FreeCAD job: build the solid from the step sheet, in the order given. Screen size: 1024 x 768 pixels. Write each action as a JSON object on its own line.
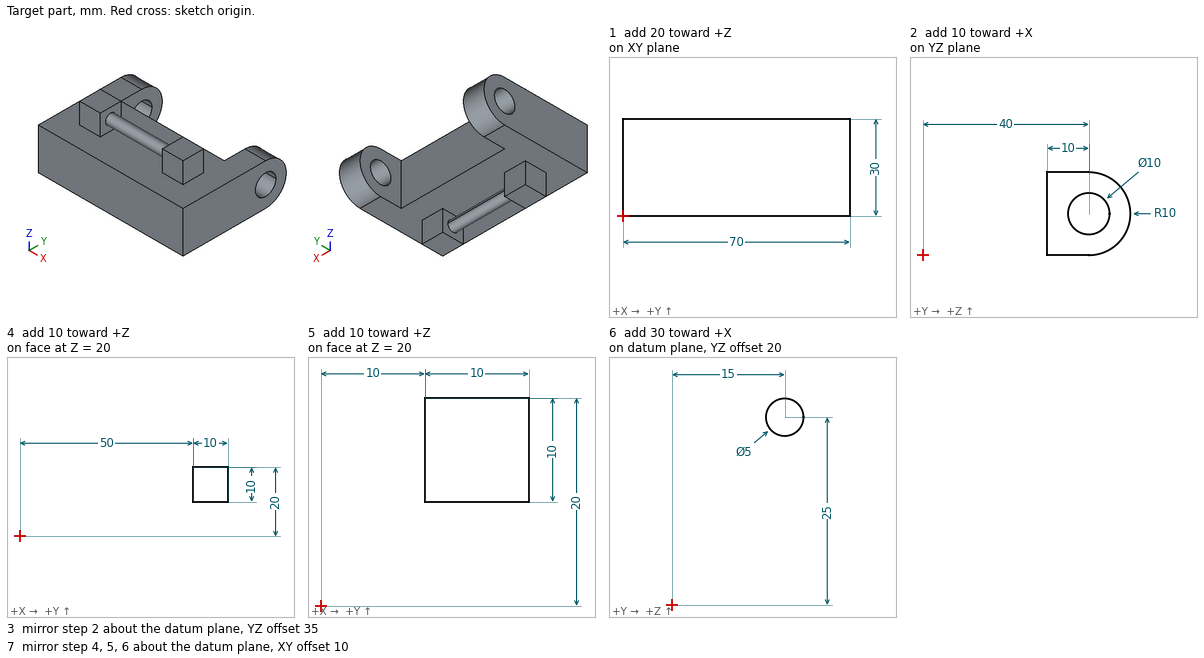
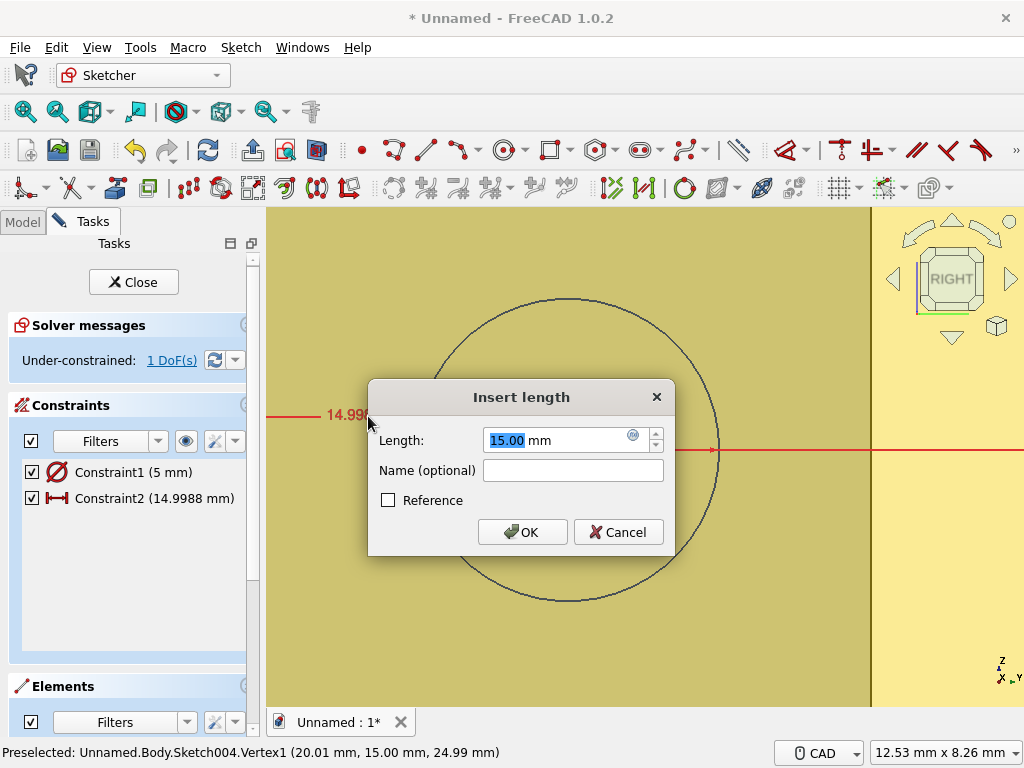
{"action": "type", "text": "15"}
{"action": "key", "text": "Return"}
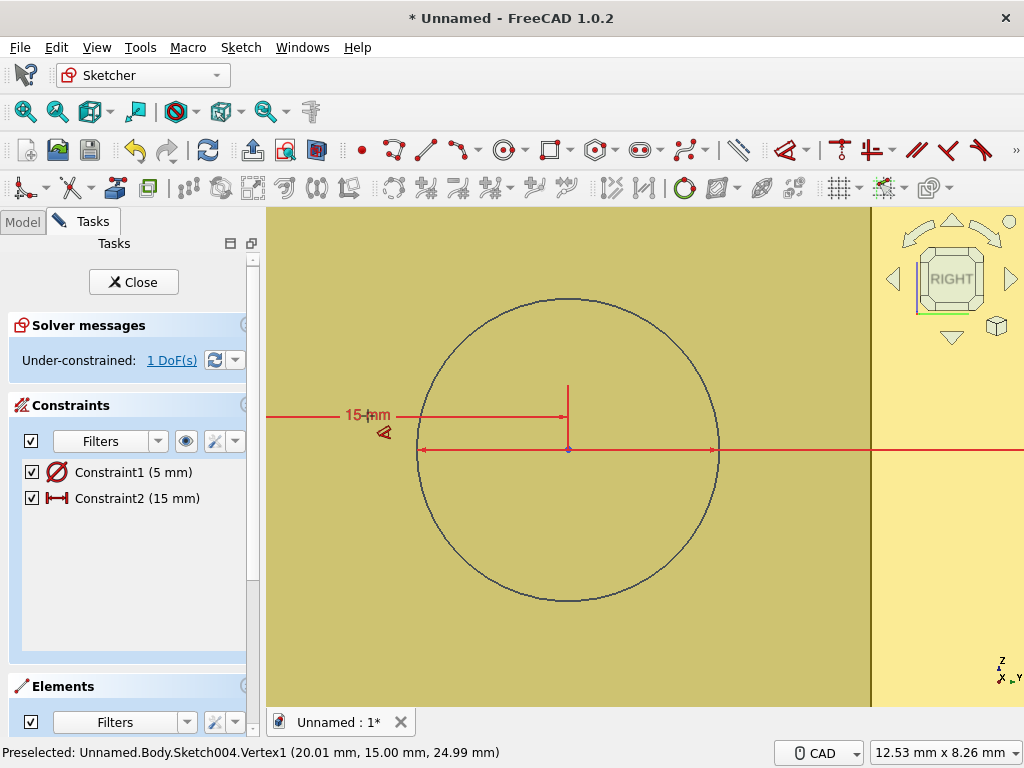
{"action": "left_click", "coordinate": [568, 450]}
{"action": "left_click", "coordinate": [602, 565]}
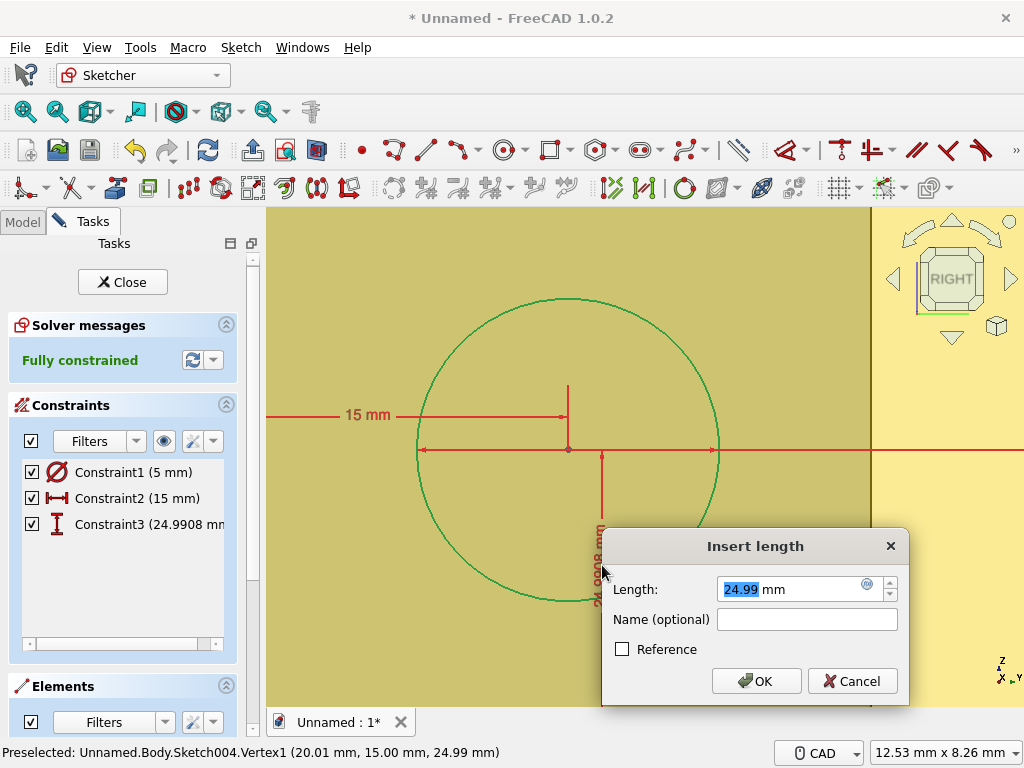
{"action": "type", "text": "25"}
{"action": "key", "text": "Return"}
{"action": "key", "text": "Escape"}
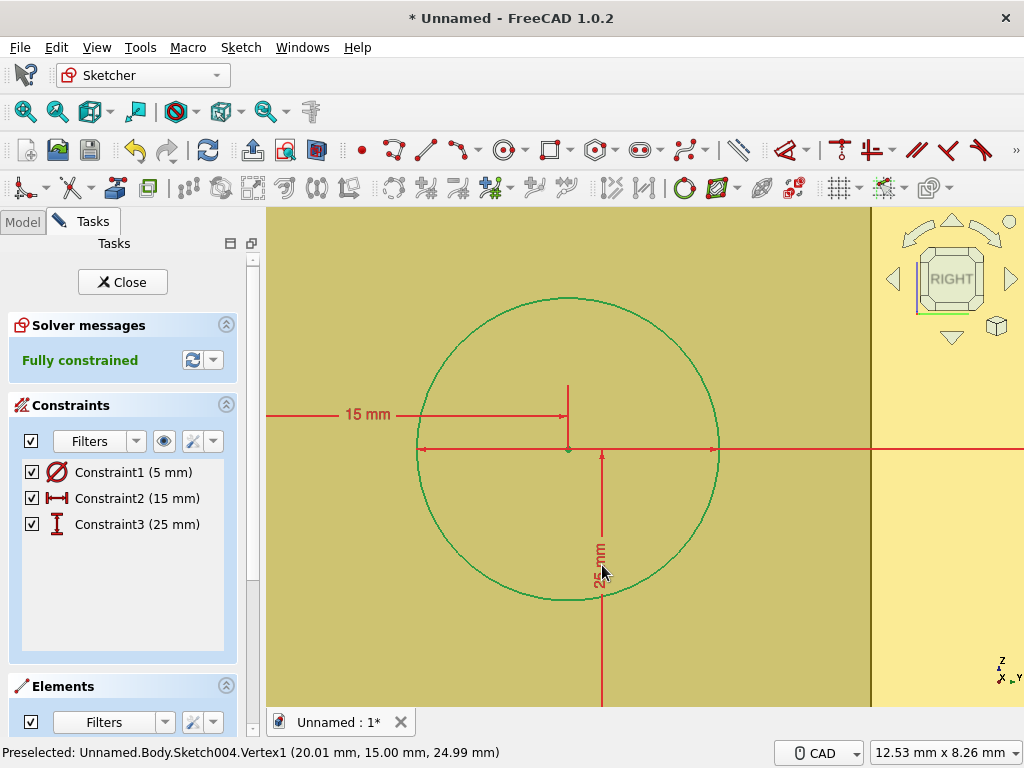
{"action": "left_click", "coordinate": [123, 282]}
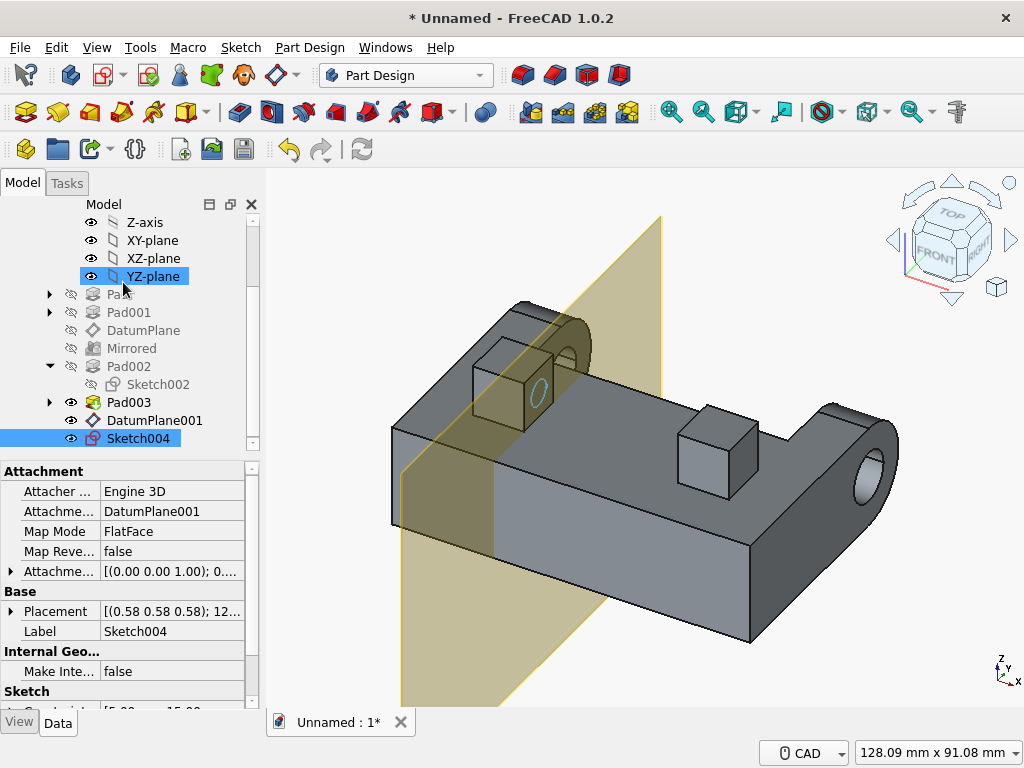
{"action": "left_click", "coordinate": [26, 112]}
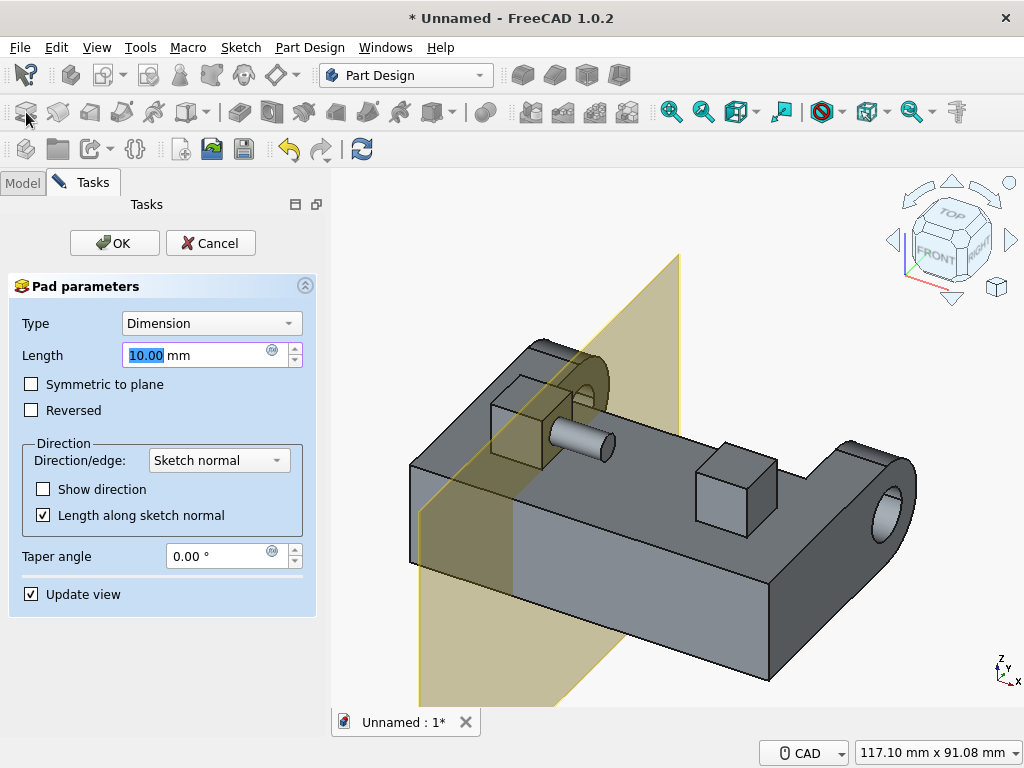
{"action": "type", "text": "30"}
{"action": "key", "text": "Tab"}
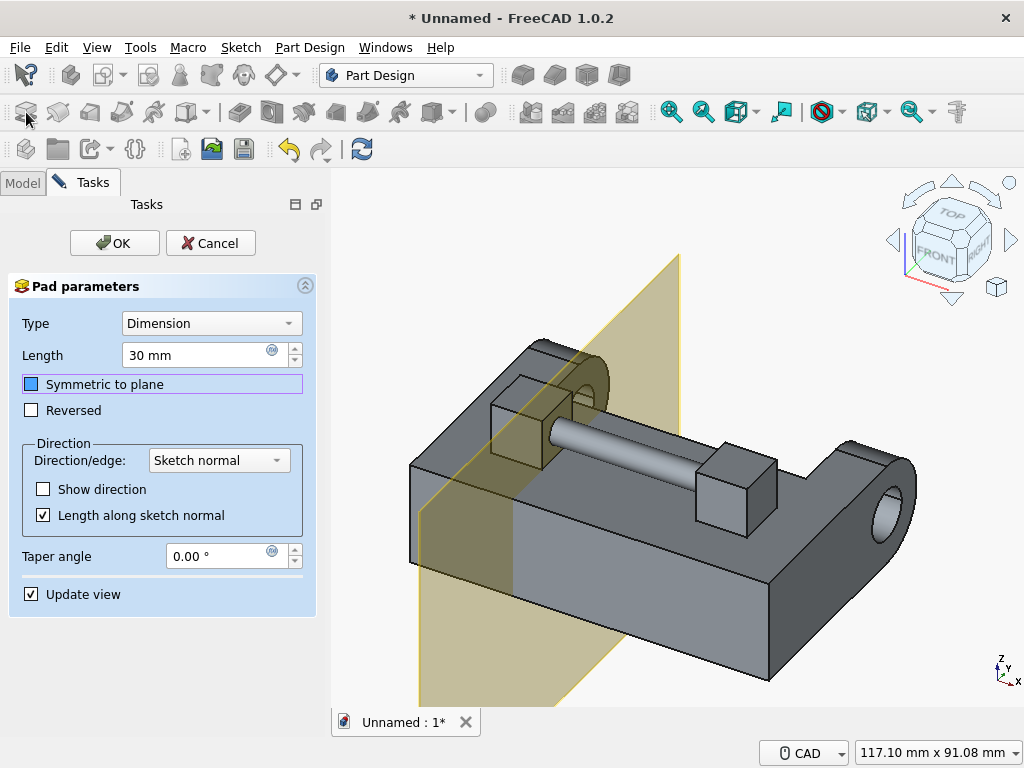
{"action": "left_click", "coordinate": [115, 243]}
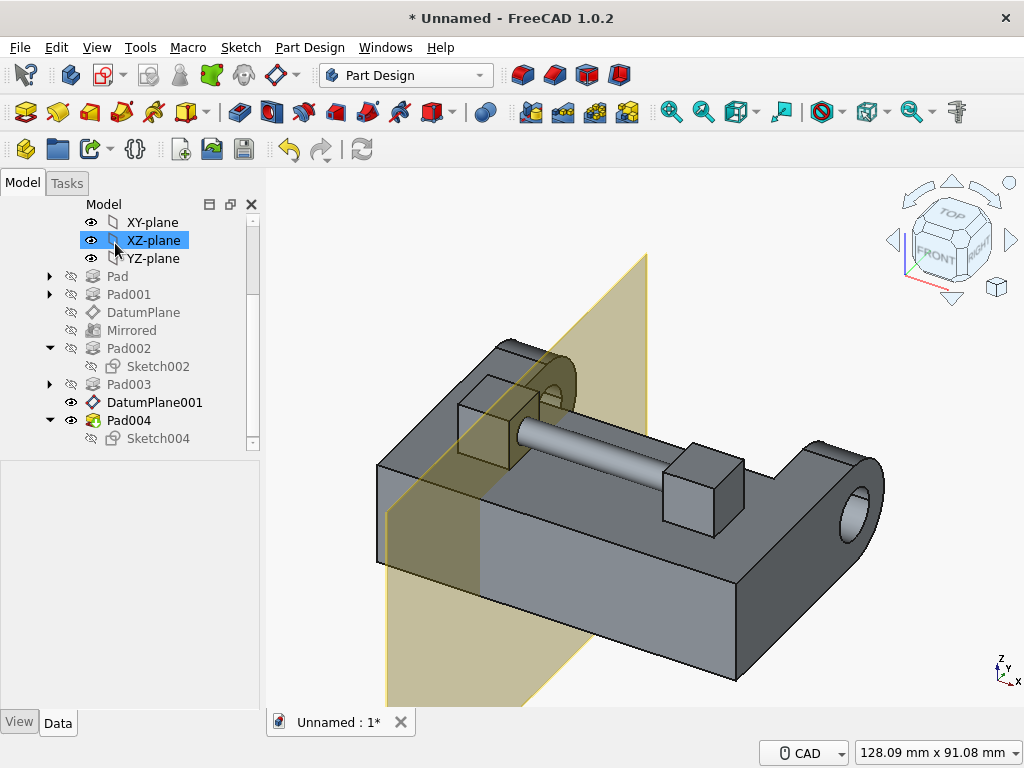
{"action": "left_click", "coordinate": [116, 402]}
{"action": "key", "text": "space"}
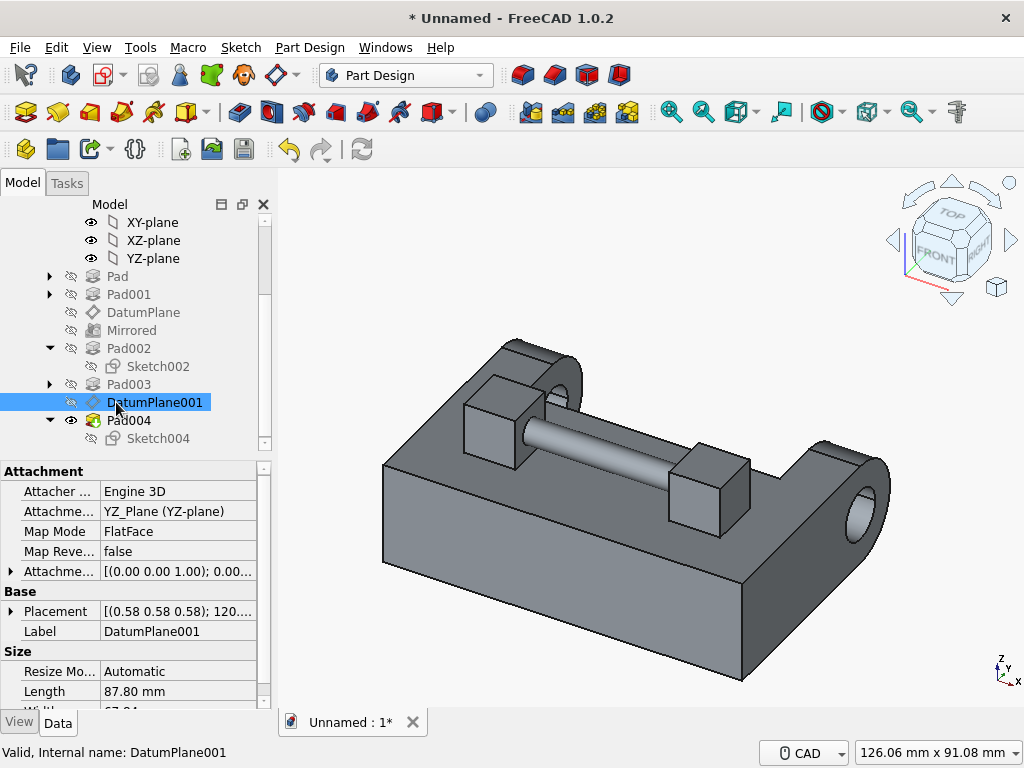
{"action": "scroll", "coordinate": [160, 326], "scroll_direction": "down", "scroll_amount": 3}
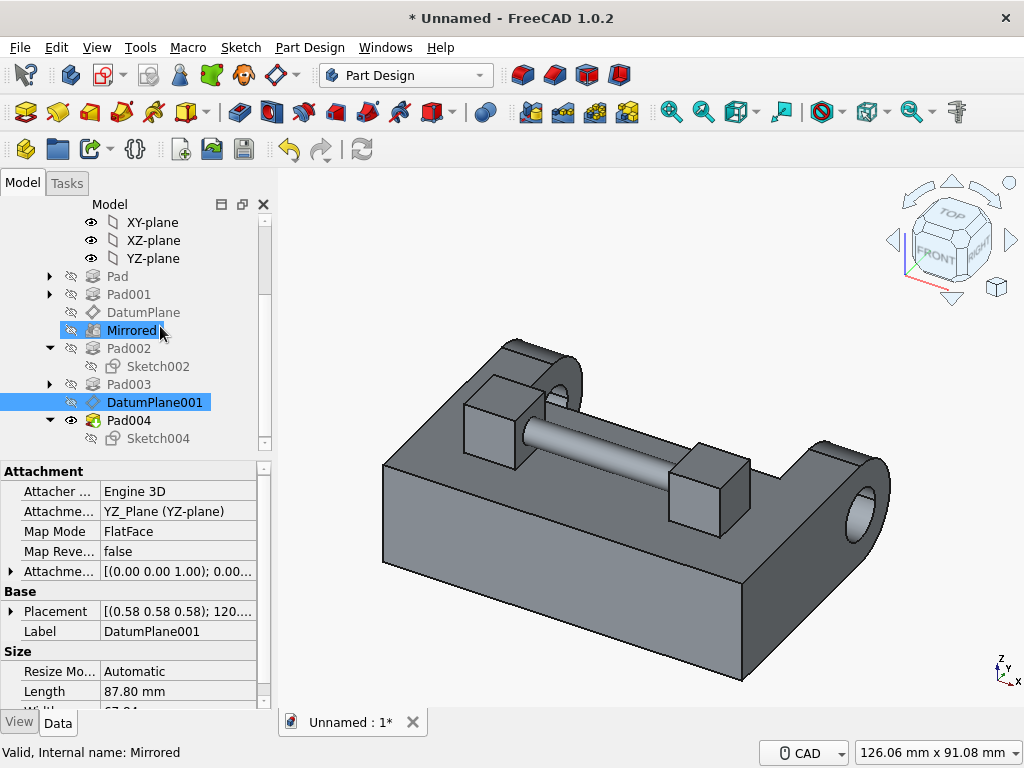
{"action": "scroll", "coordinate": [160, 326], "scroll_direction": "up", "scroll_amount": 15}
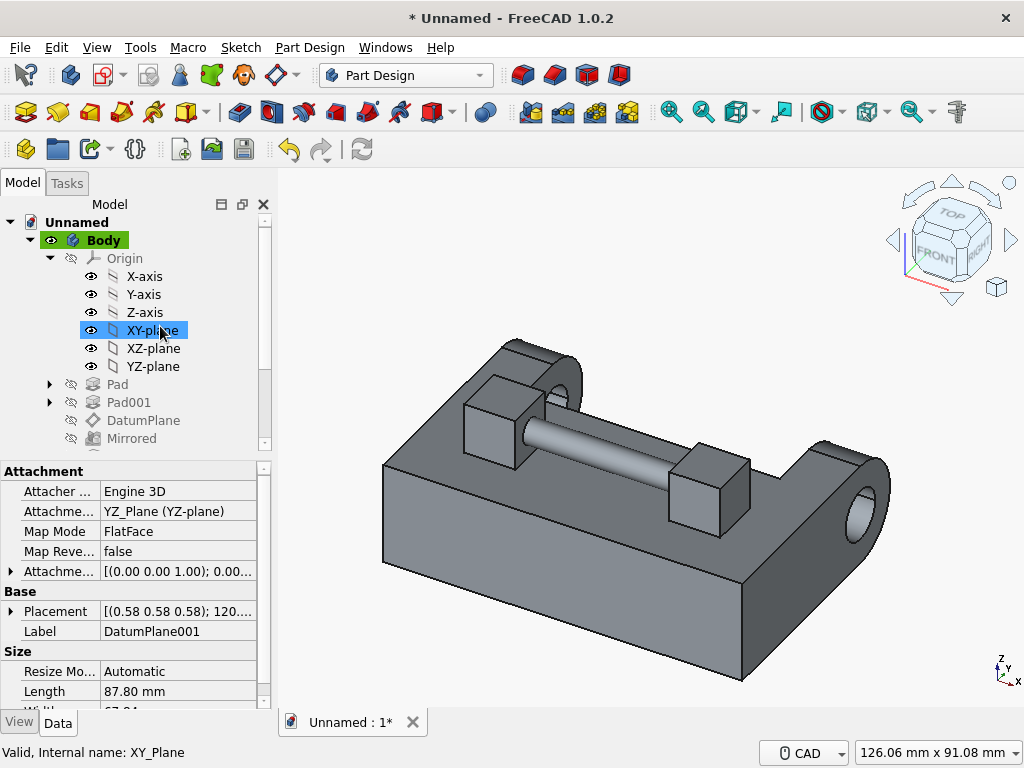
{"action": "left_click", "coordinate": [136, 330]}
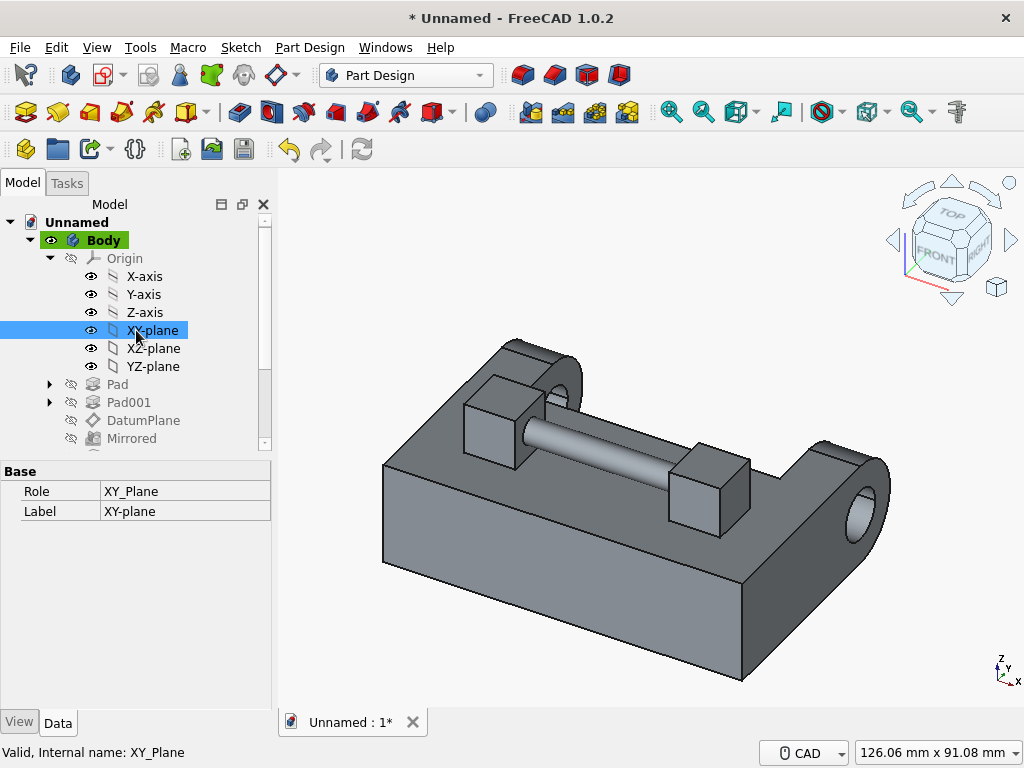
{"action": "left_click", "coordinate": [276, 76]}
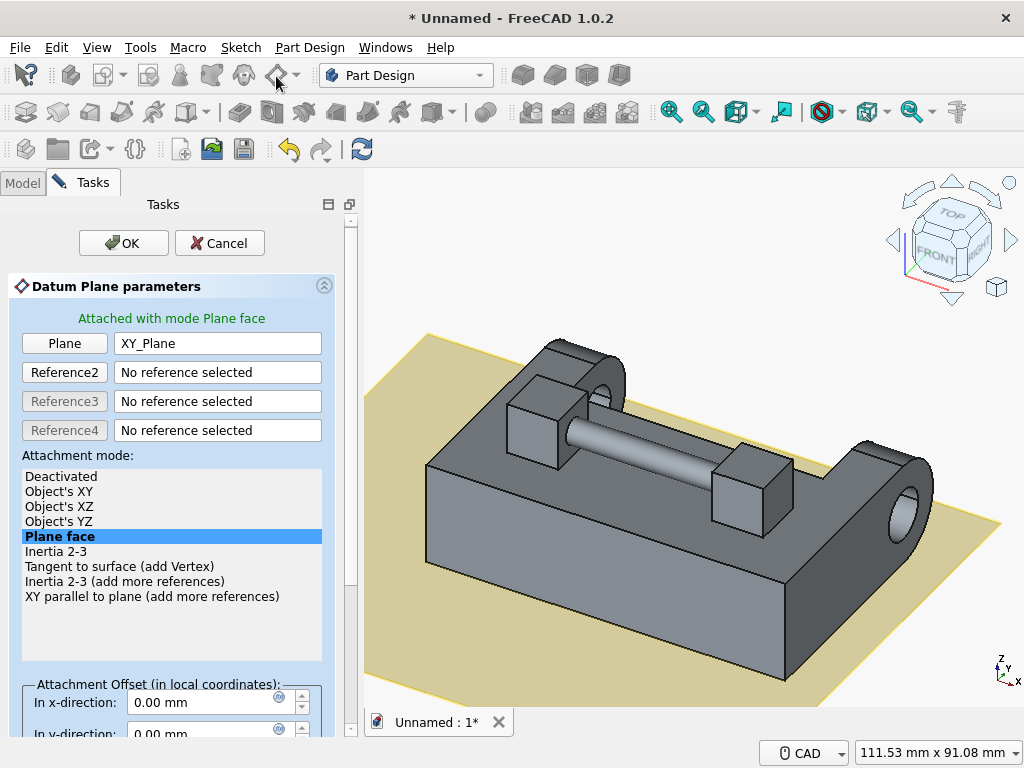
{"action": "scroll", "coordinate": [351, 475], "scroll_direction": "down", "scroll_amount": 2}